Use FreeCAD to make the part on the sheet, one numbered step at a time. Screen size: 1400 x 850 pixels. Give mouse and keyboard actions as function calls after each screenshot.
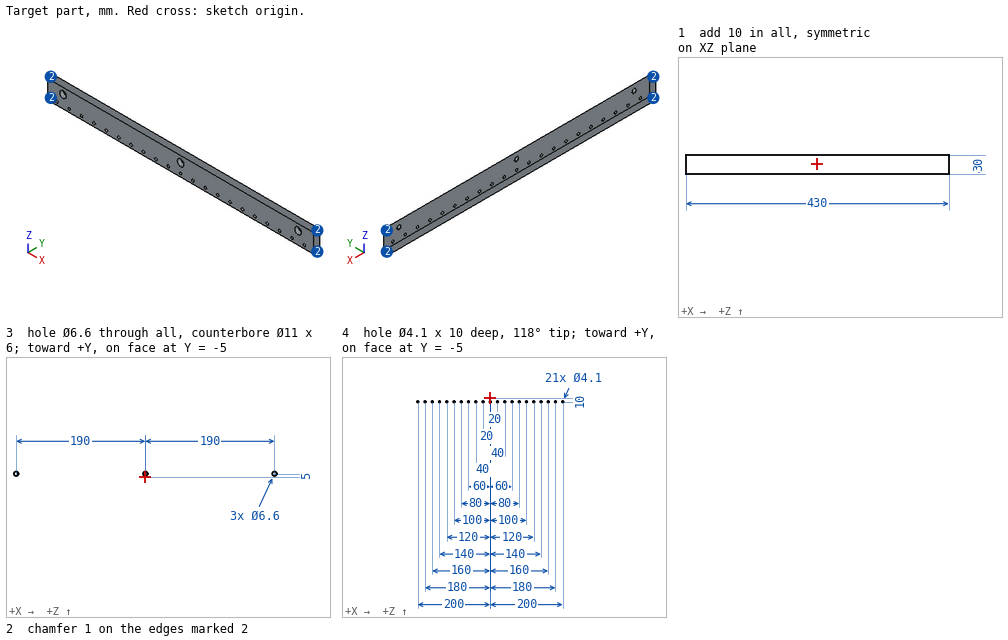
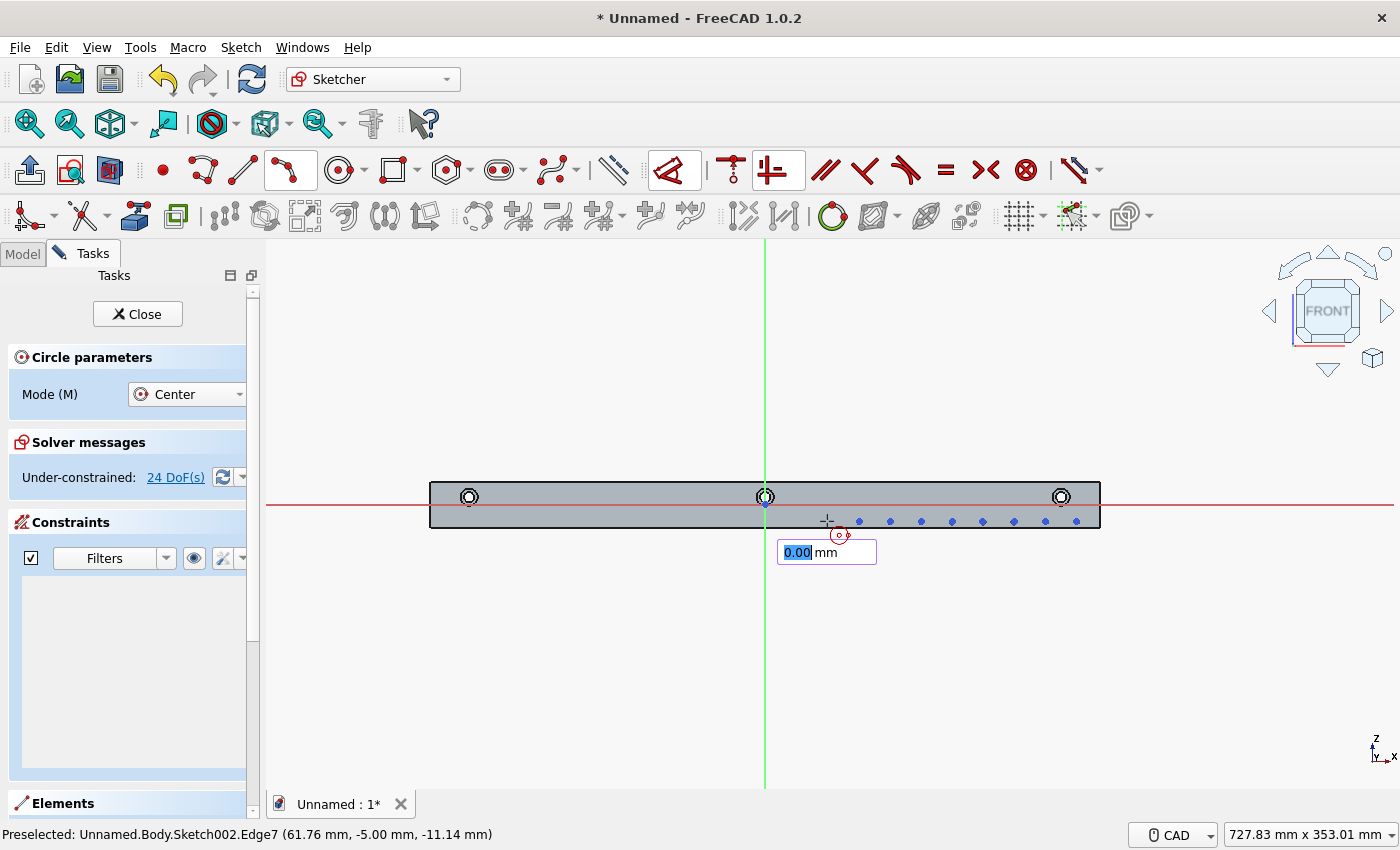
scroll(830, 523, up, 9)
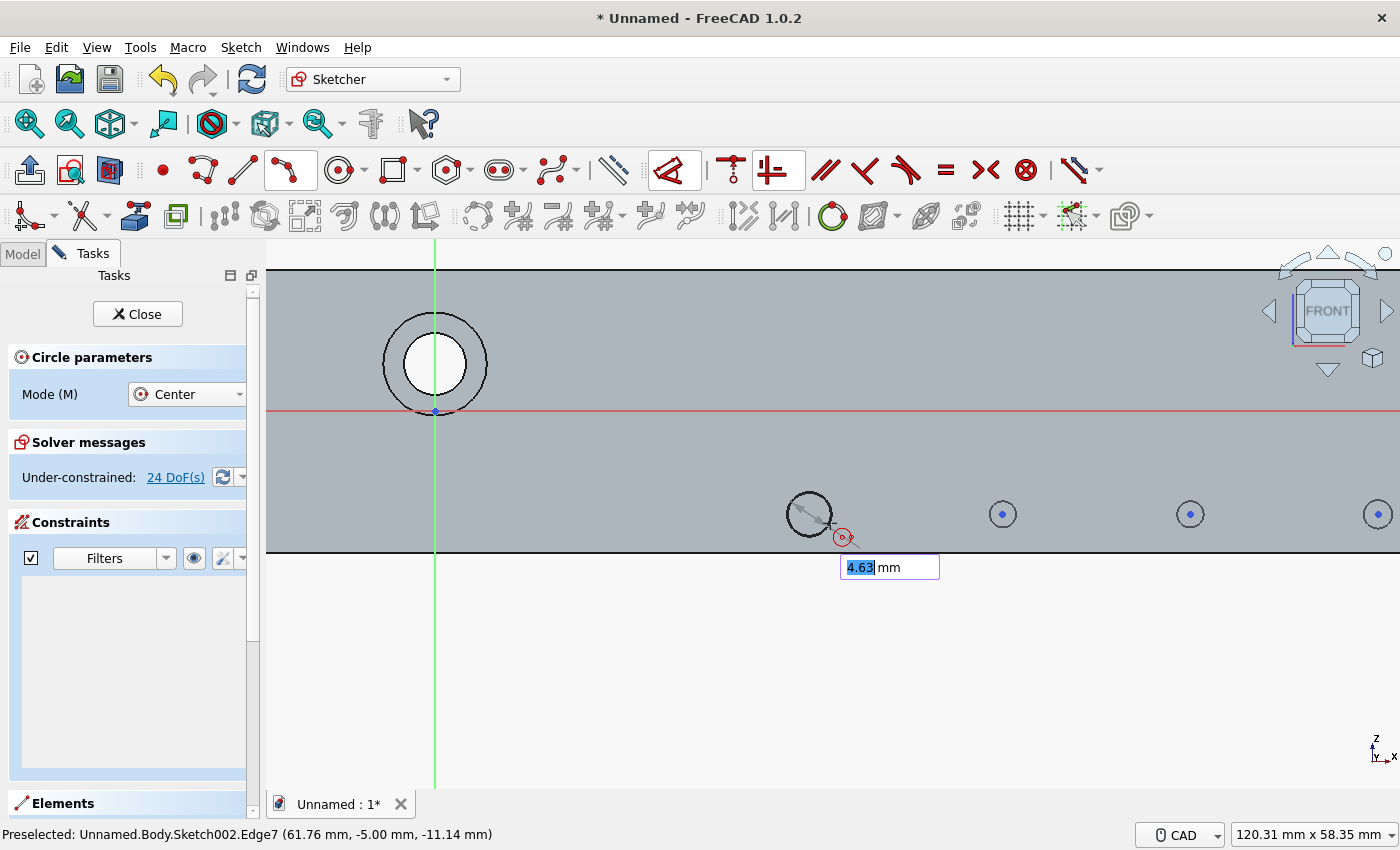
click(826, 519)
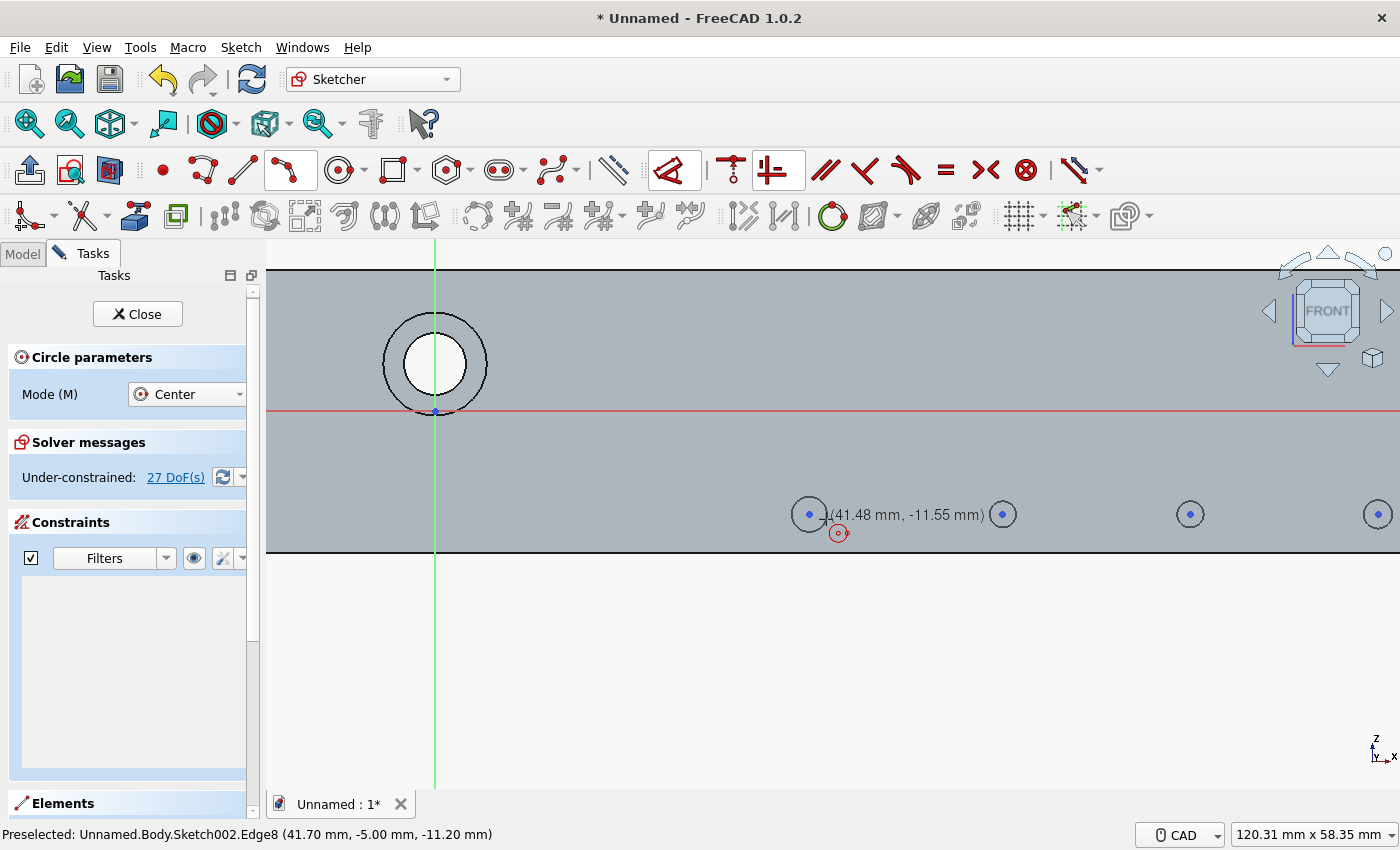
scroll(830, 523, down, 9)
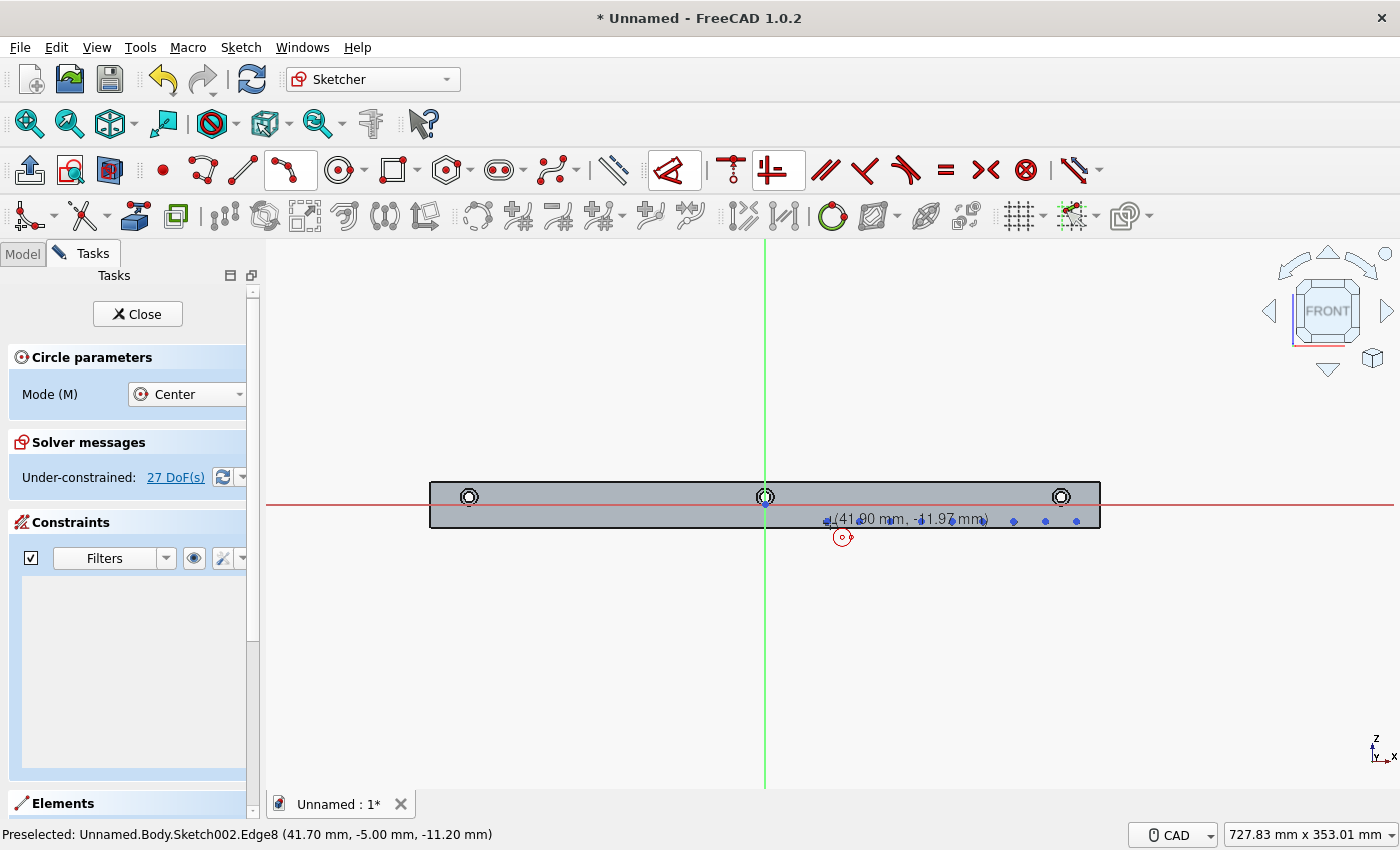
click(796, 521)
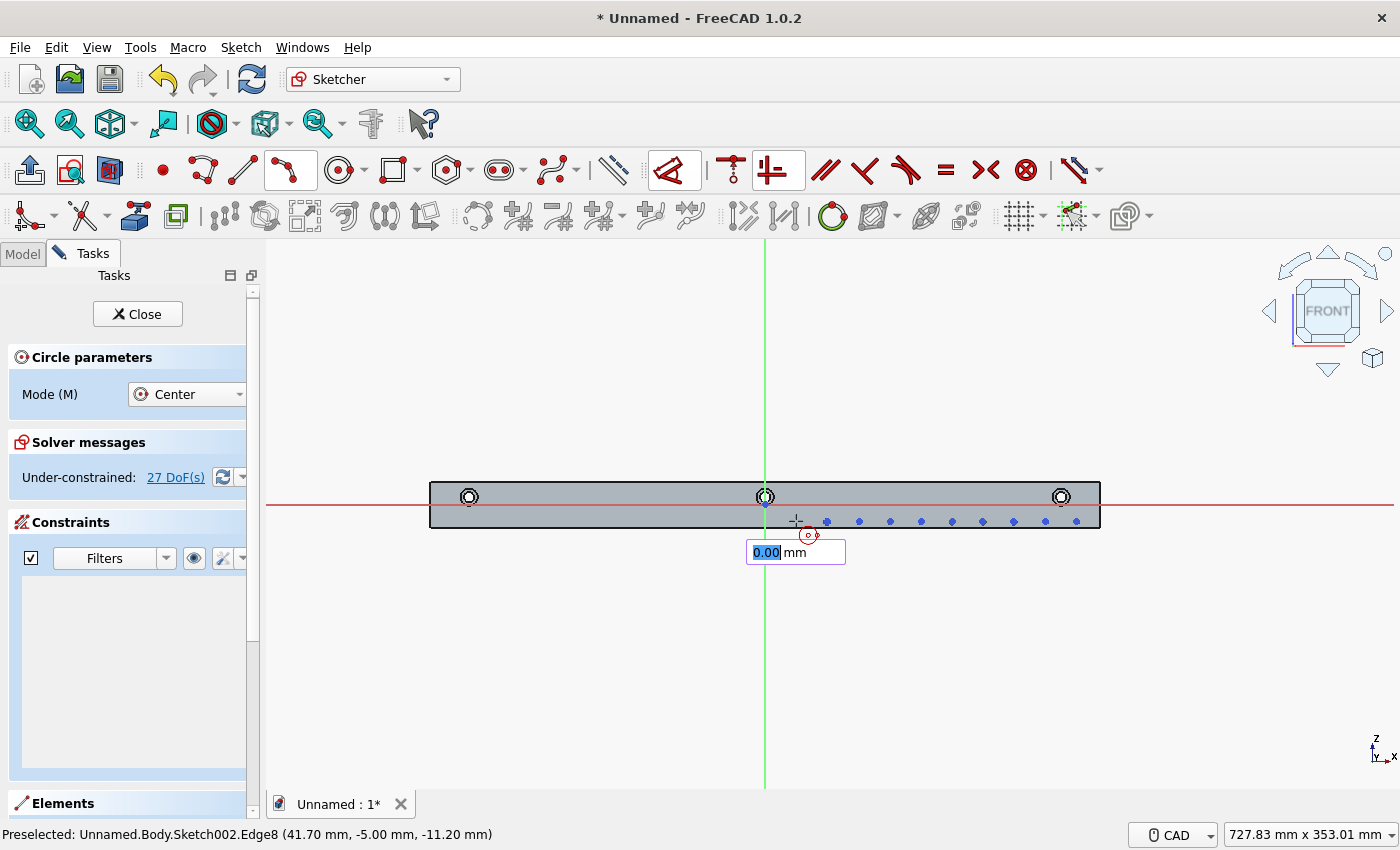
scroll(799, 523, up, 9)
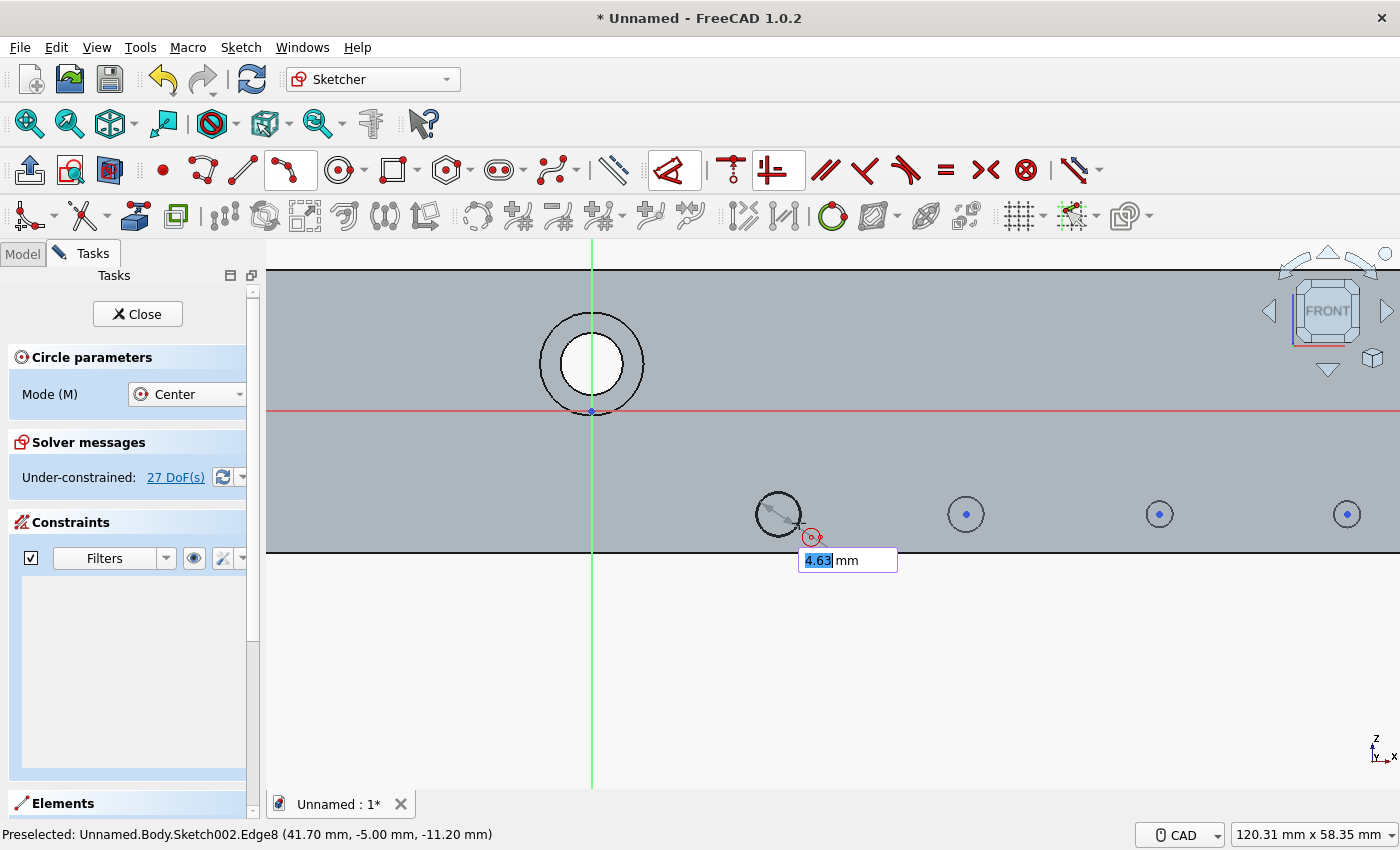
click(794, 519)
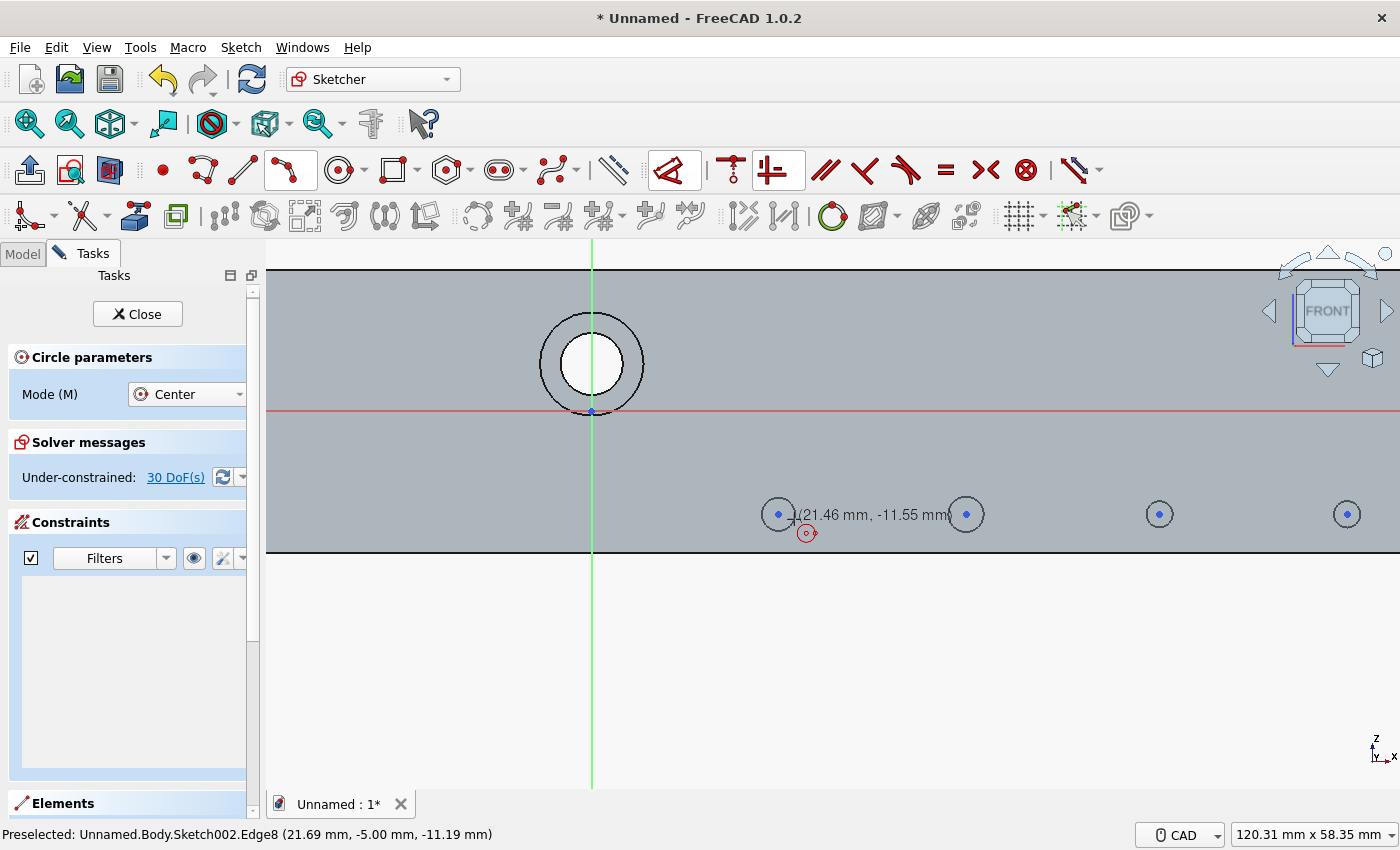
scroll(799, 523, down, 9)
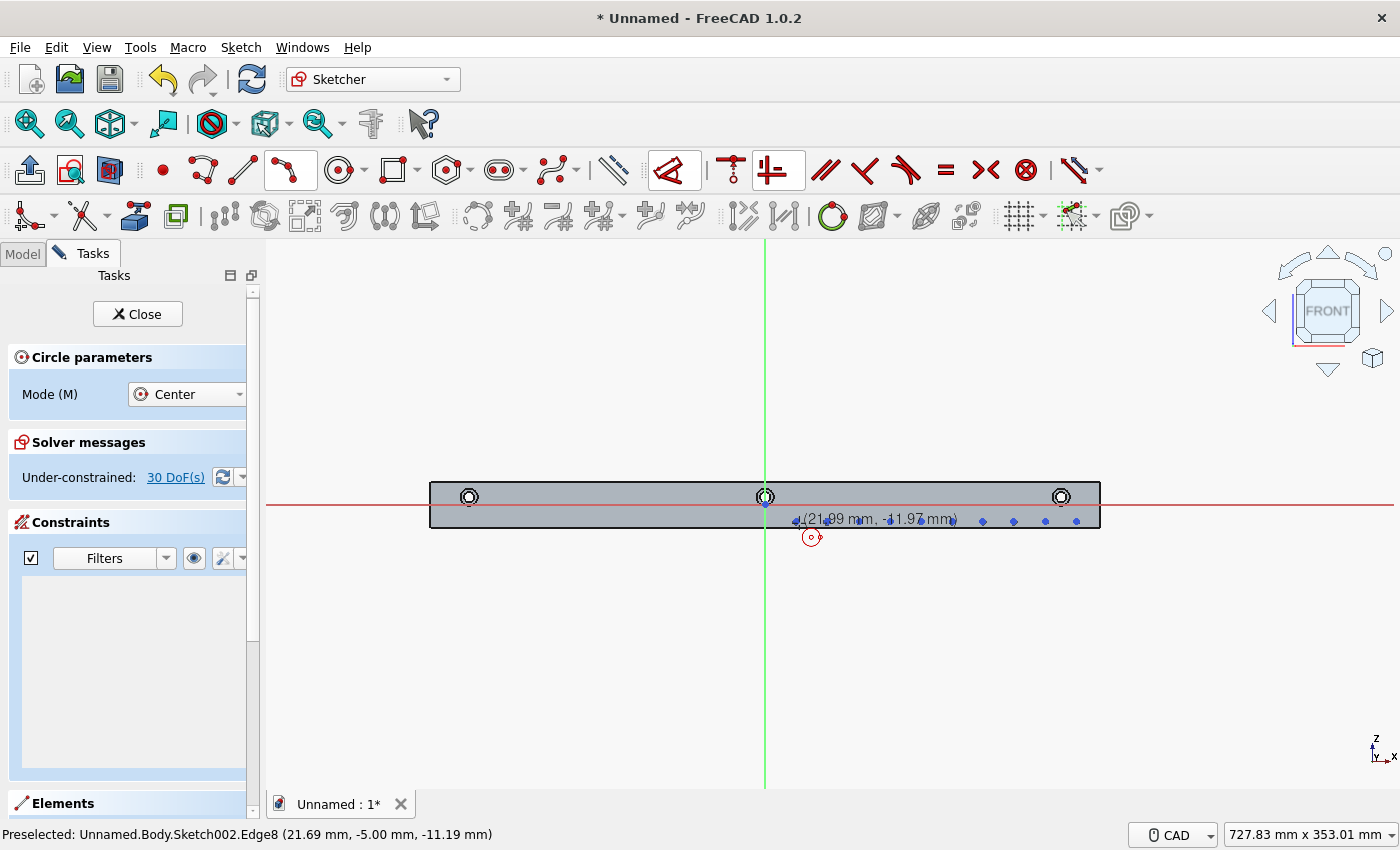
click(765, 521)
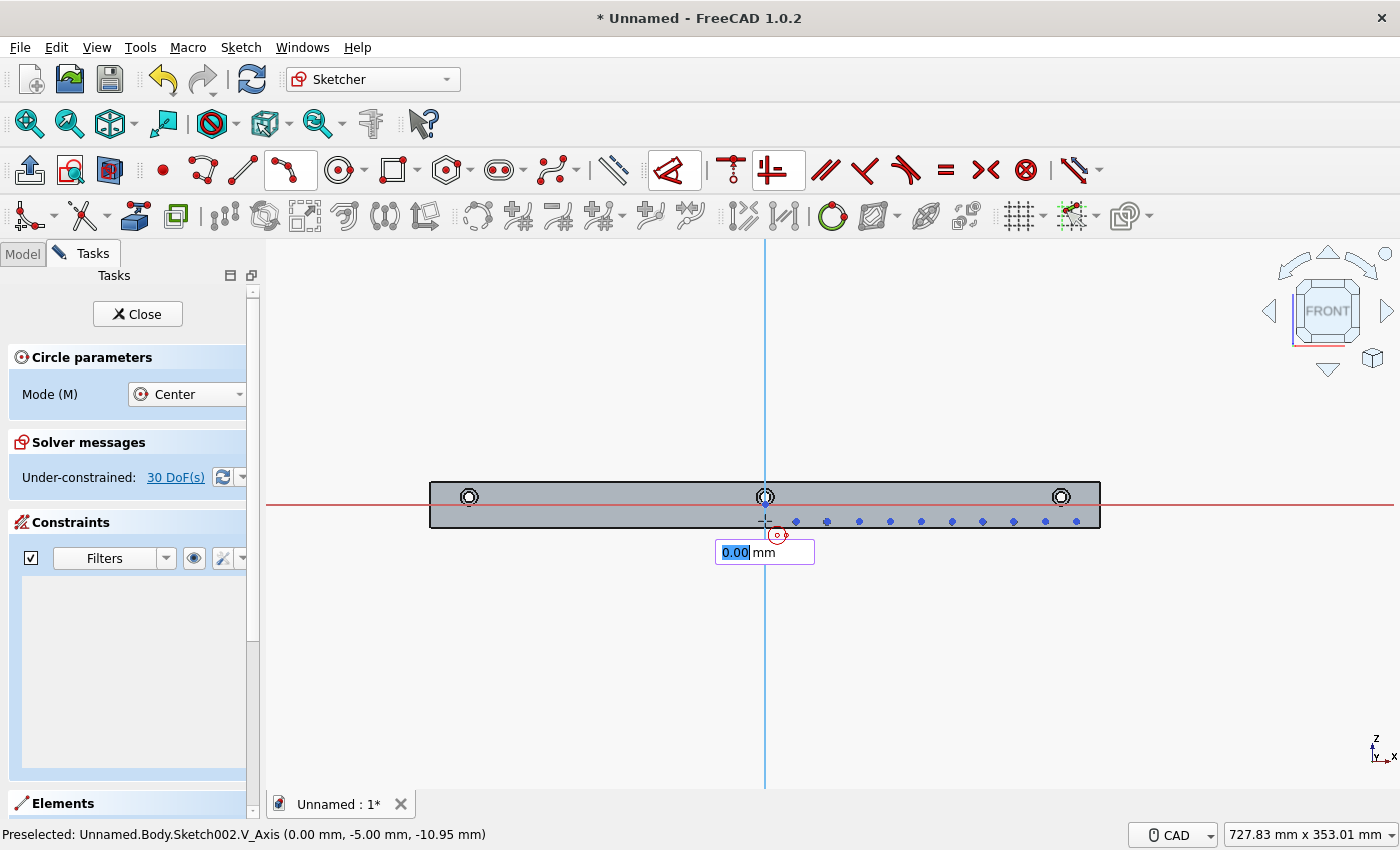
scroll(768, 519, up, 9)